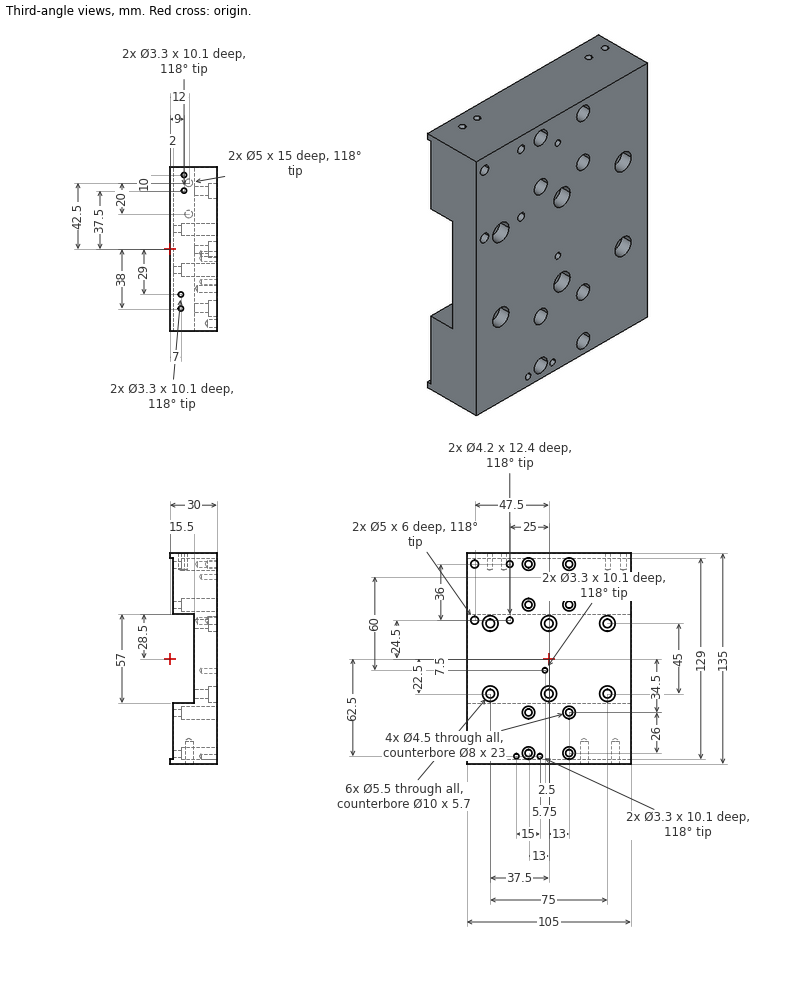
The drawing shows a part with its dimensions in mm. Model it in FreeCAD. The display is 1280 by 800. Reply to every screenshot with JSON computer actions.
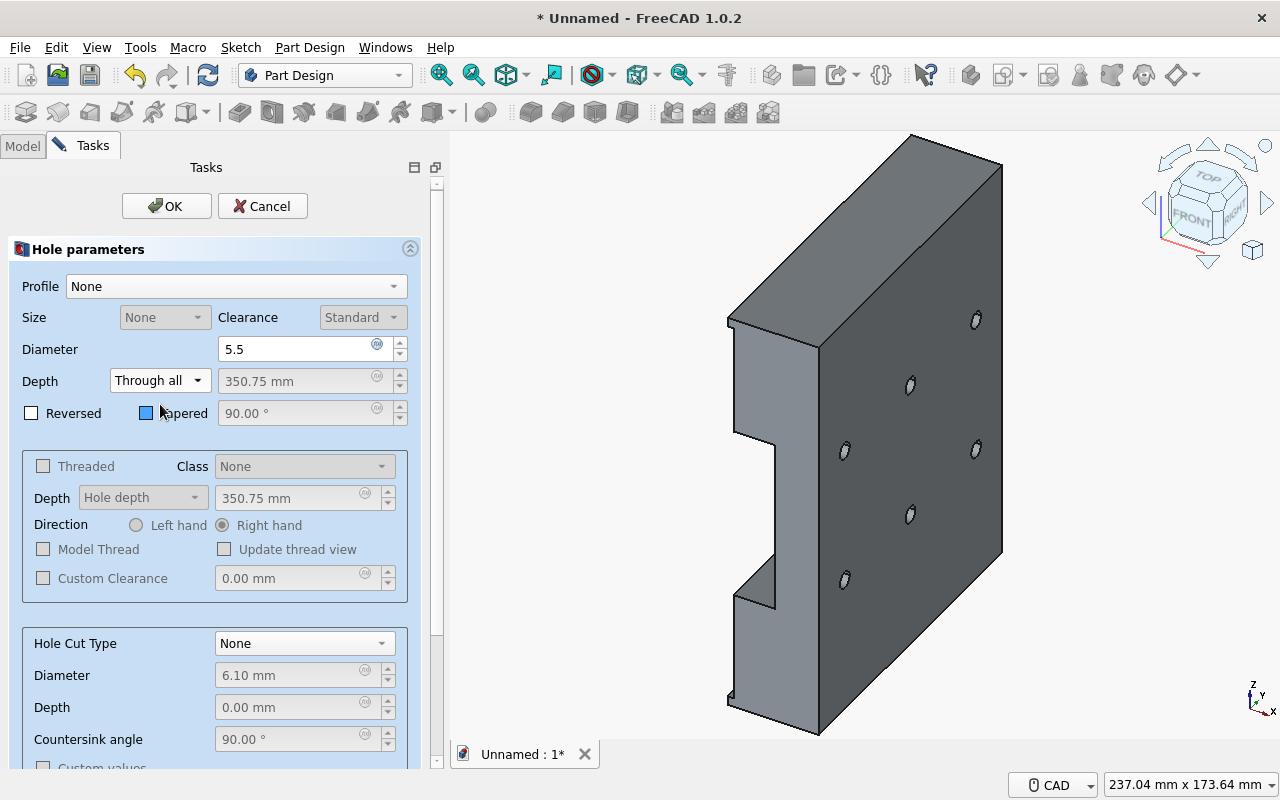
{"action": "left_click", "coordinate": [306, 644]}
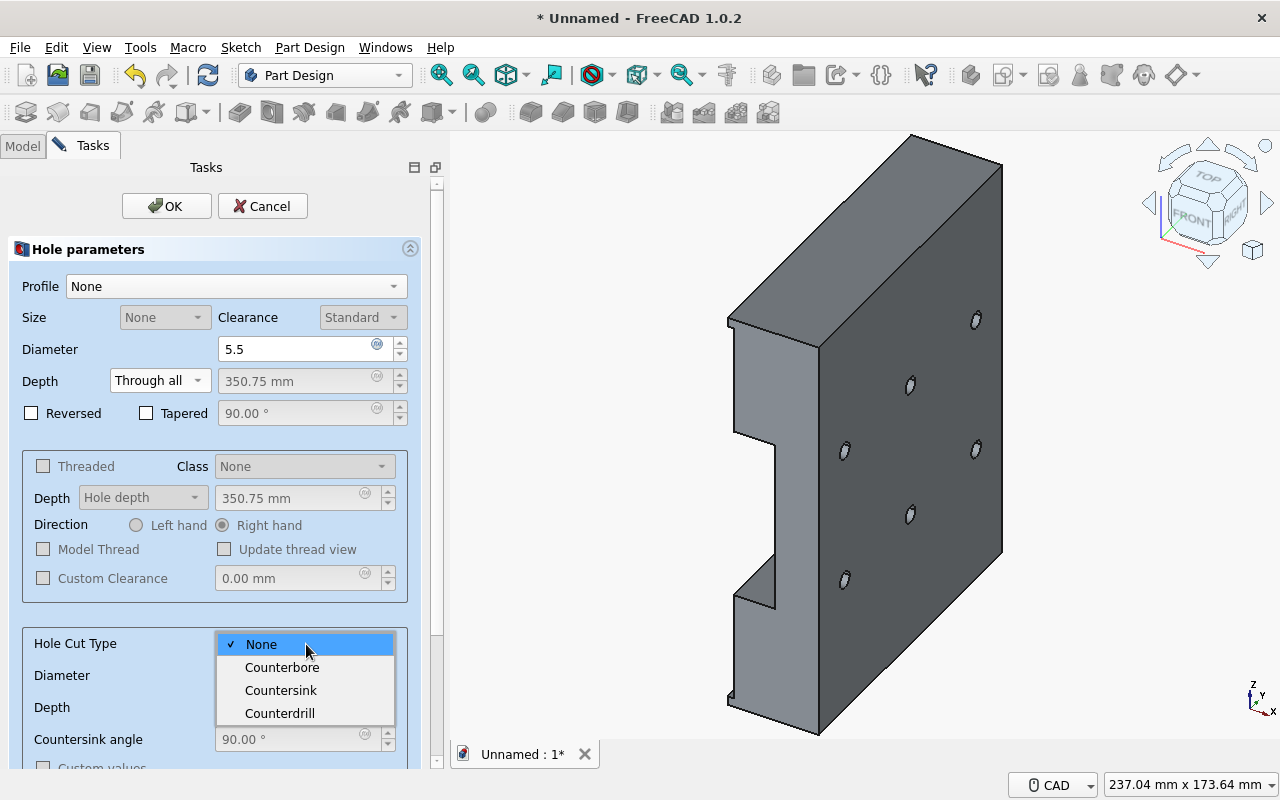
{"action": "left_click", "coordinate": [304, 668]}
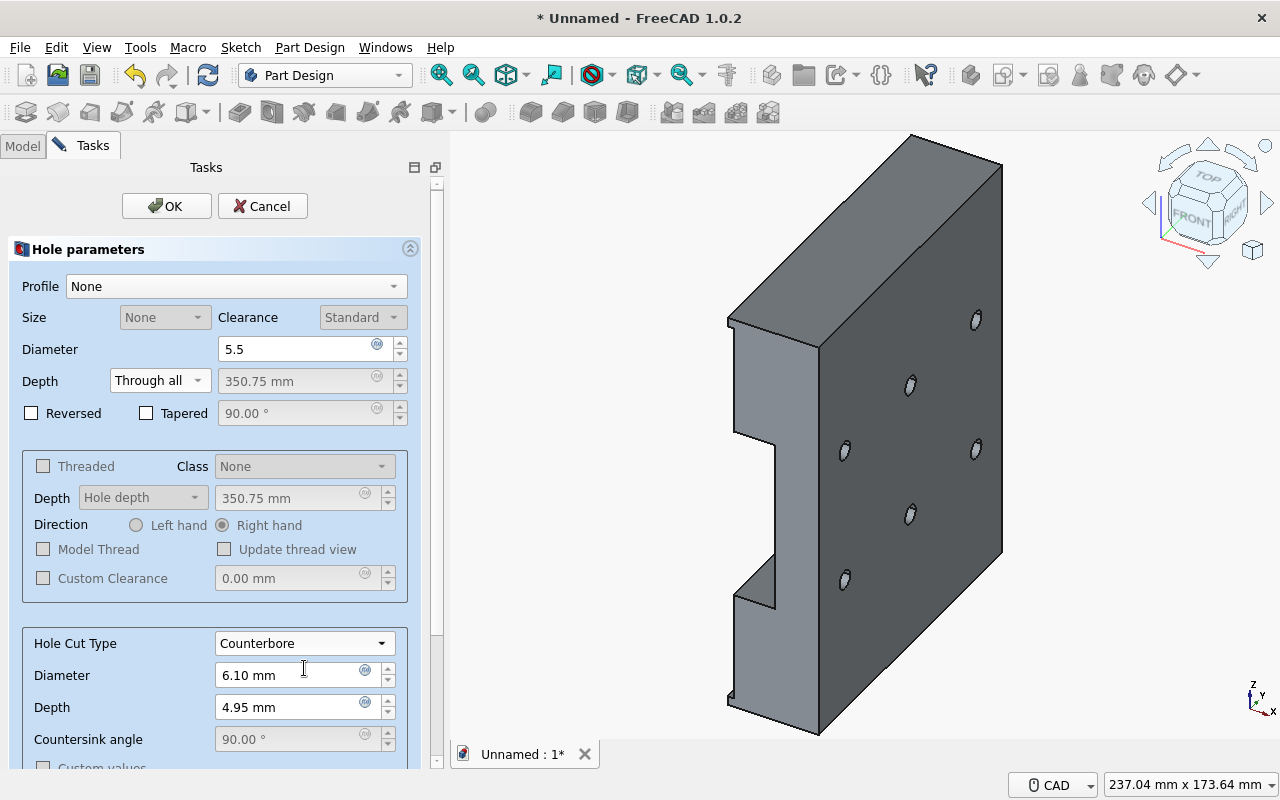
{"action": "triple_click", "coordinate": [298, 675]}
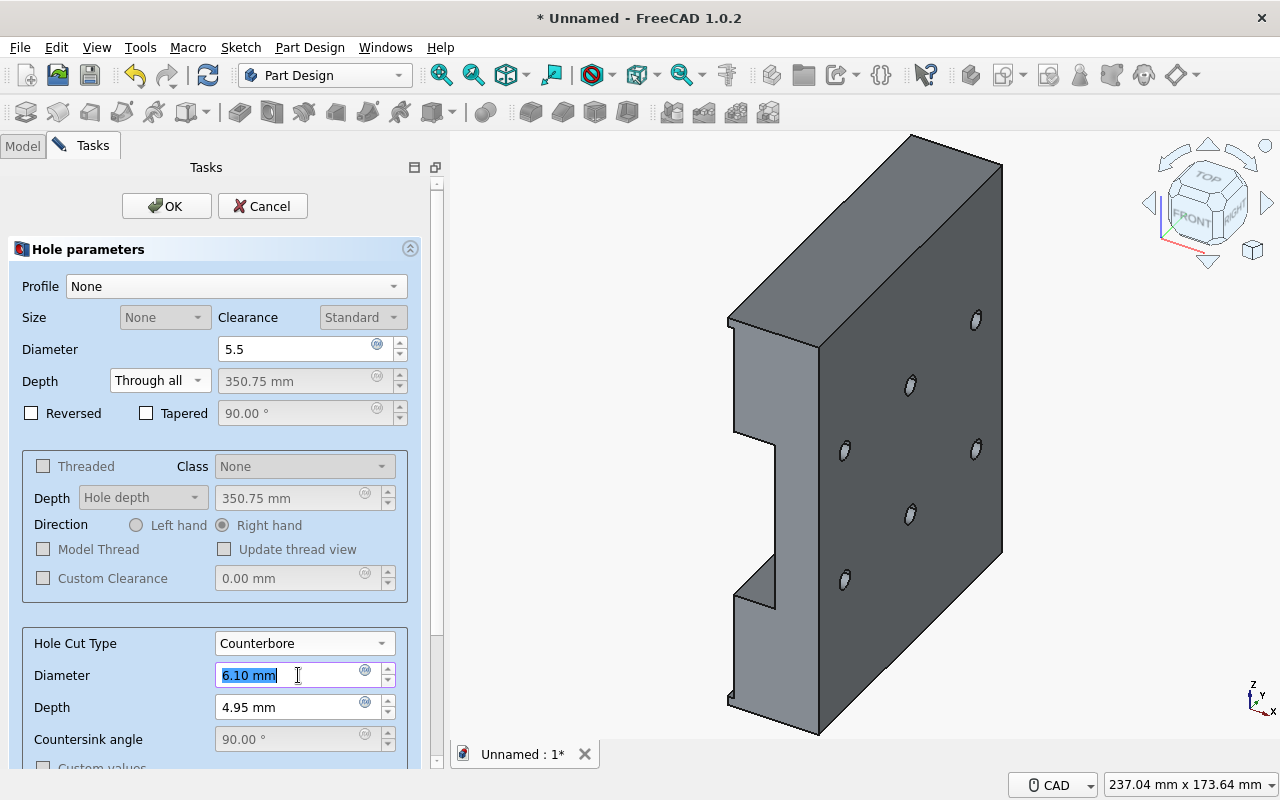
{"action": "type", "text": "10"}
{"action": "key", "text": "Tab"}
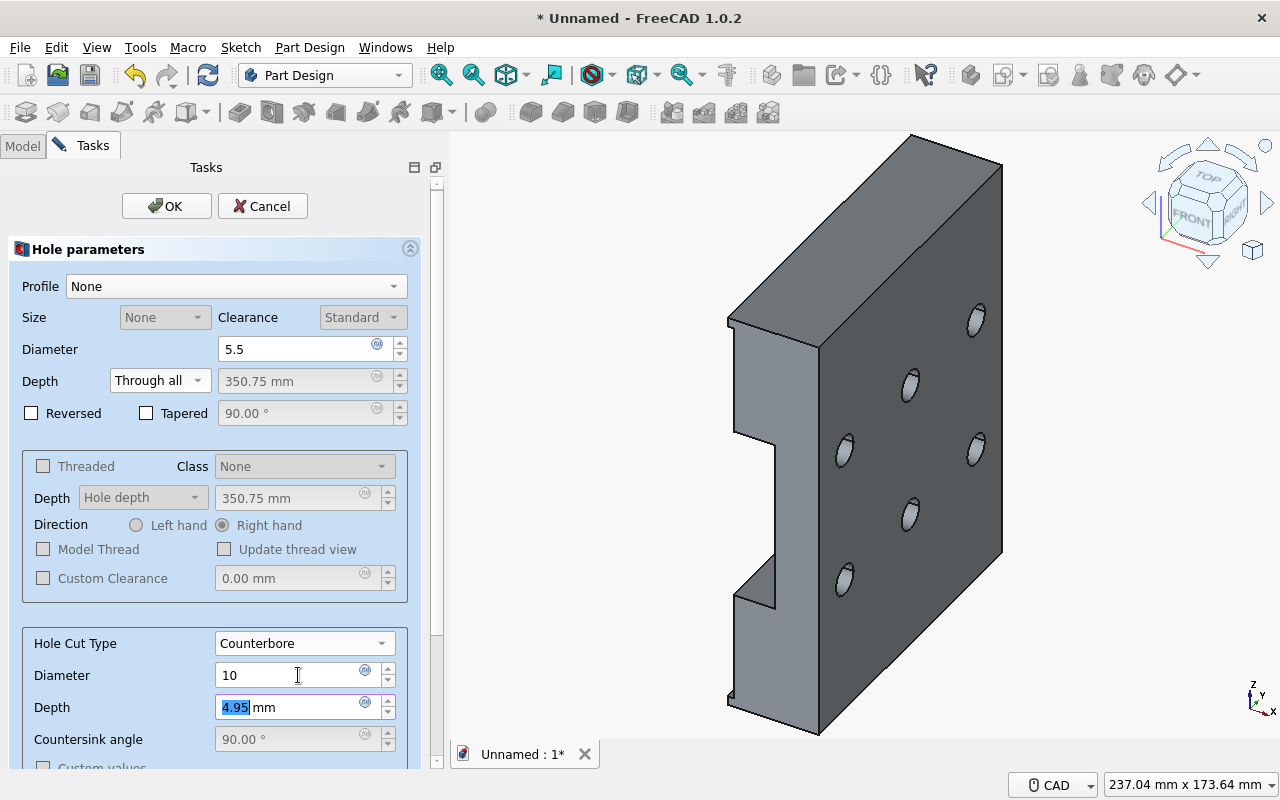
{"action": "type", "text": "5.7"}
{"action": "key", "text": "Tab"}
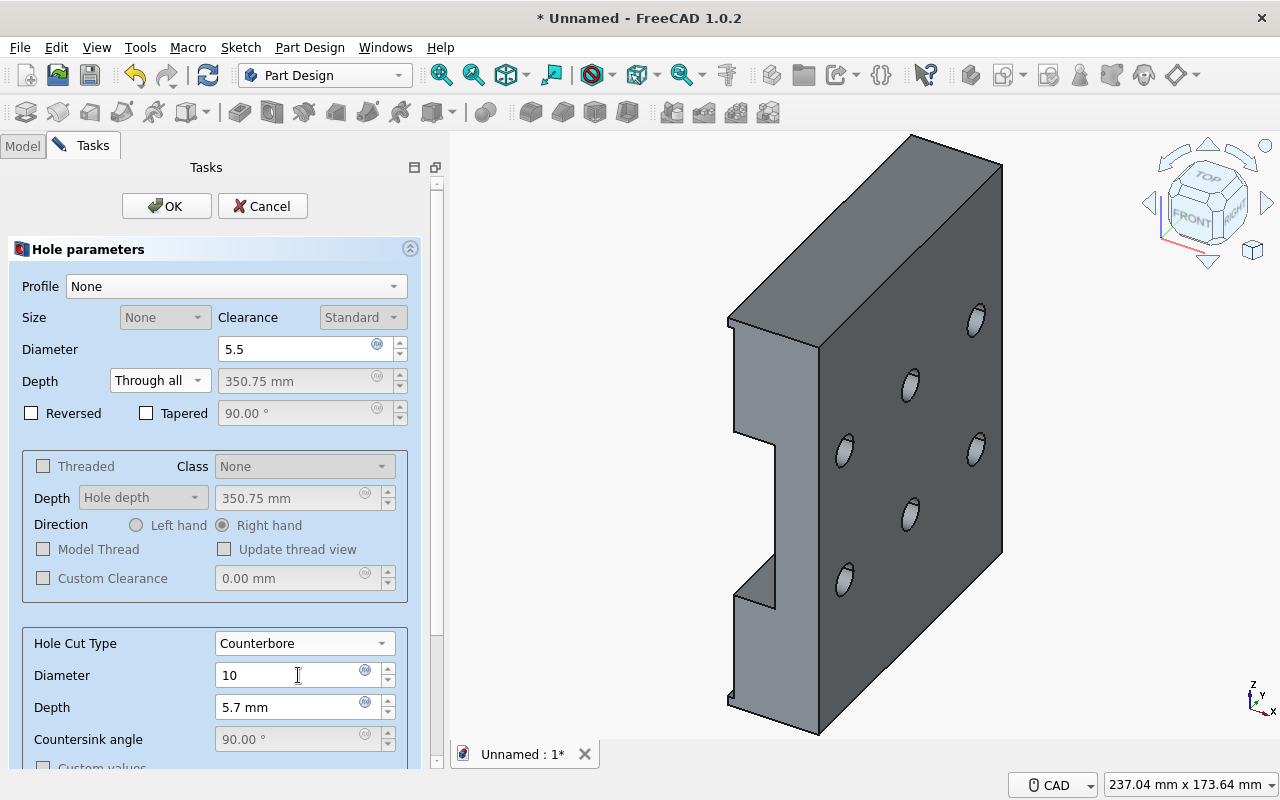
{"action": "left_click", "coordinate": [167, 206]}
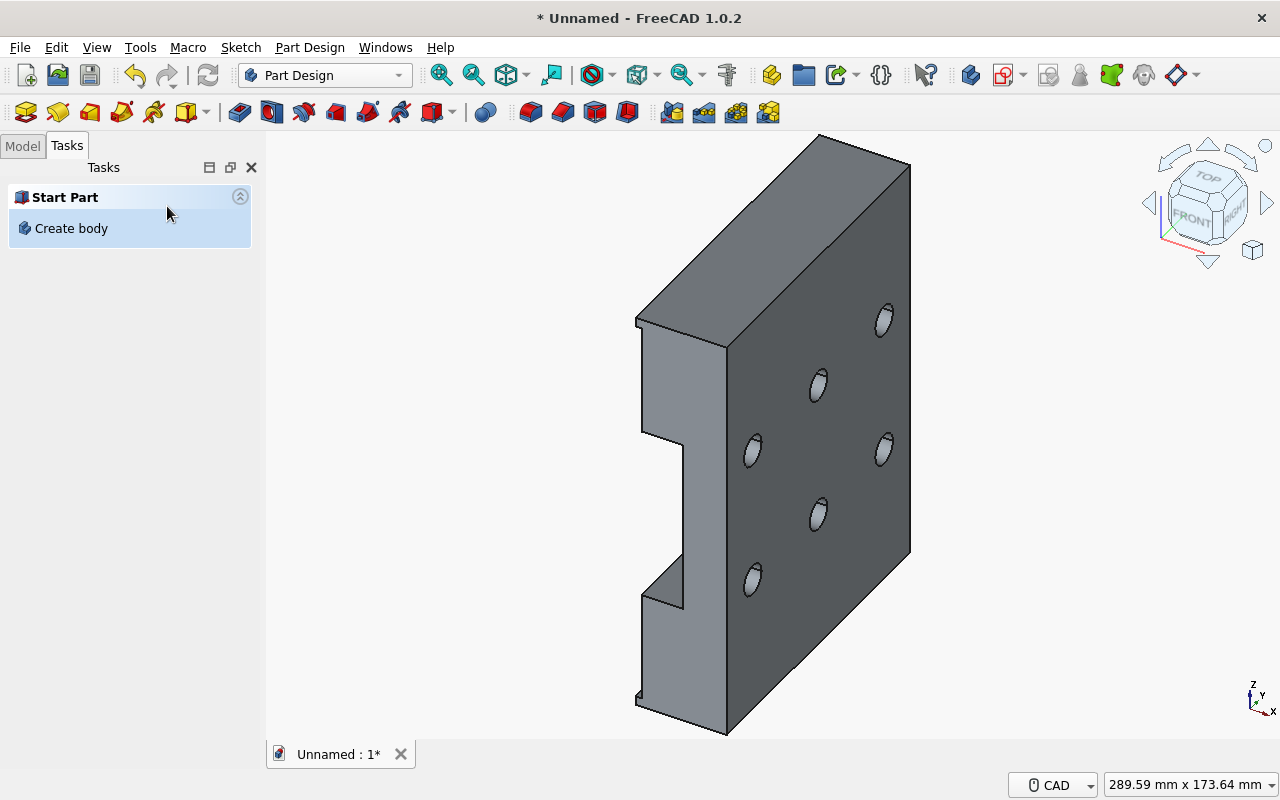
{"action": "left_click", "coordinate": [792, 475]}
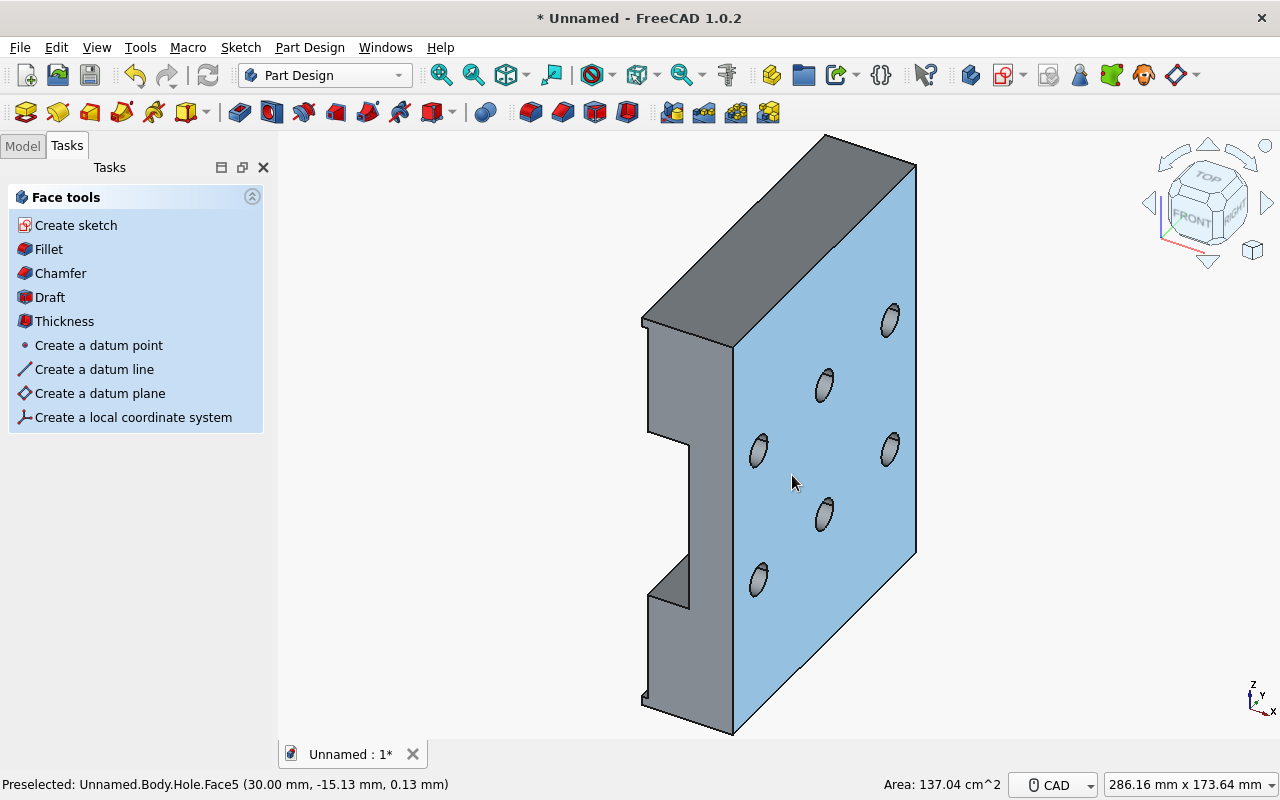
{"action": "left_click", "coordinate": [1004, 76]}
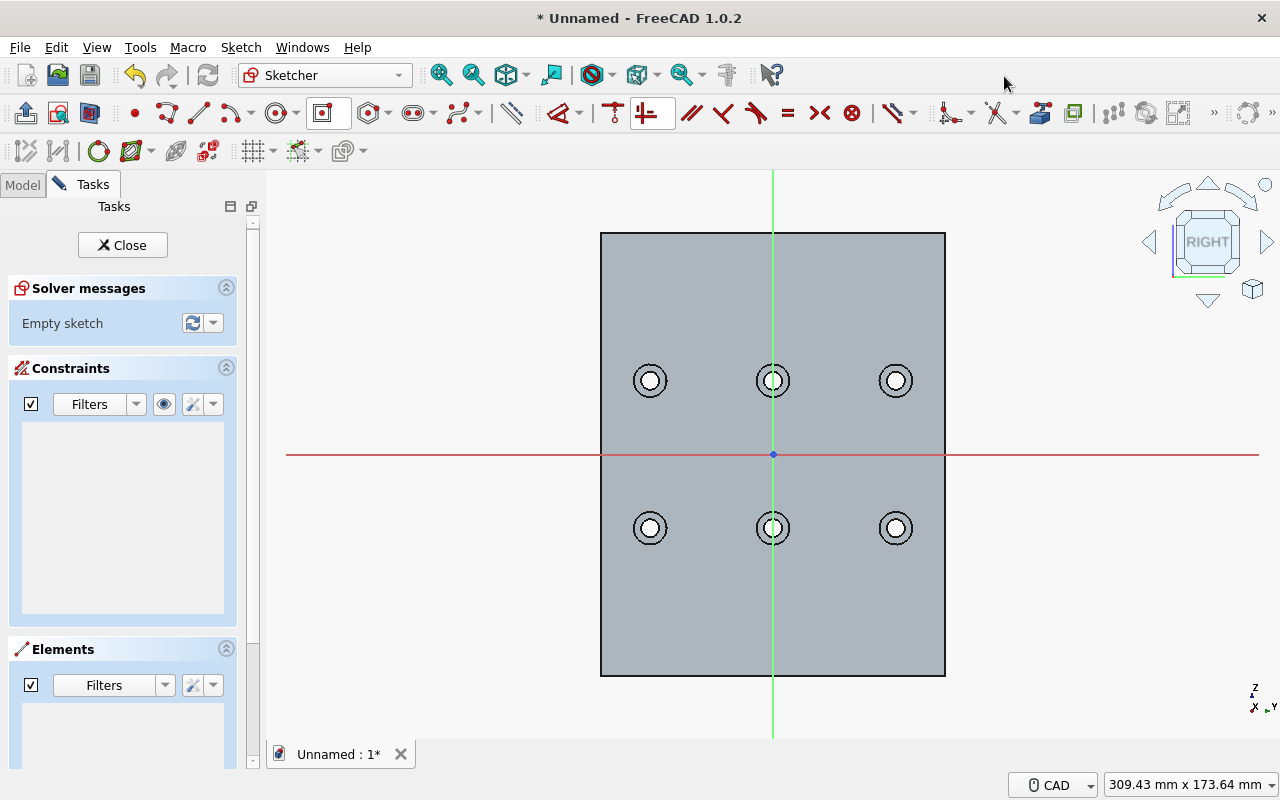
{"action": "scroll", "coordinate": [856, 682], "scroll_direction": "up", "scroll_amount": 3}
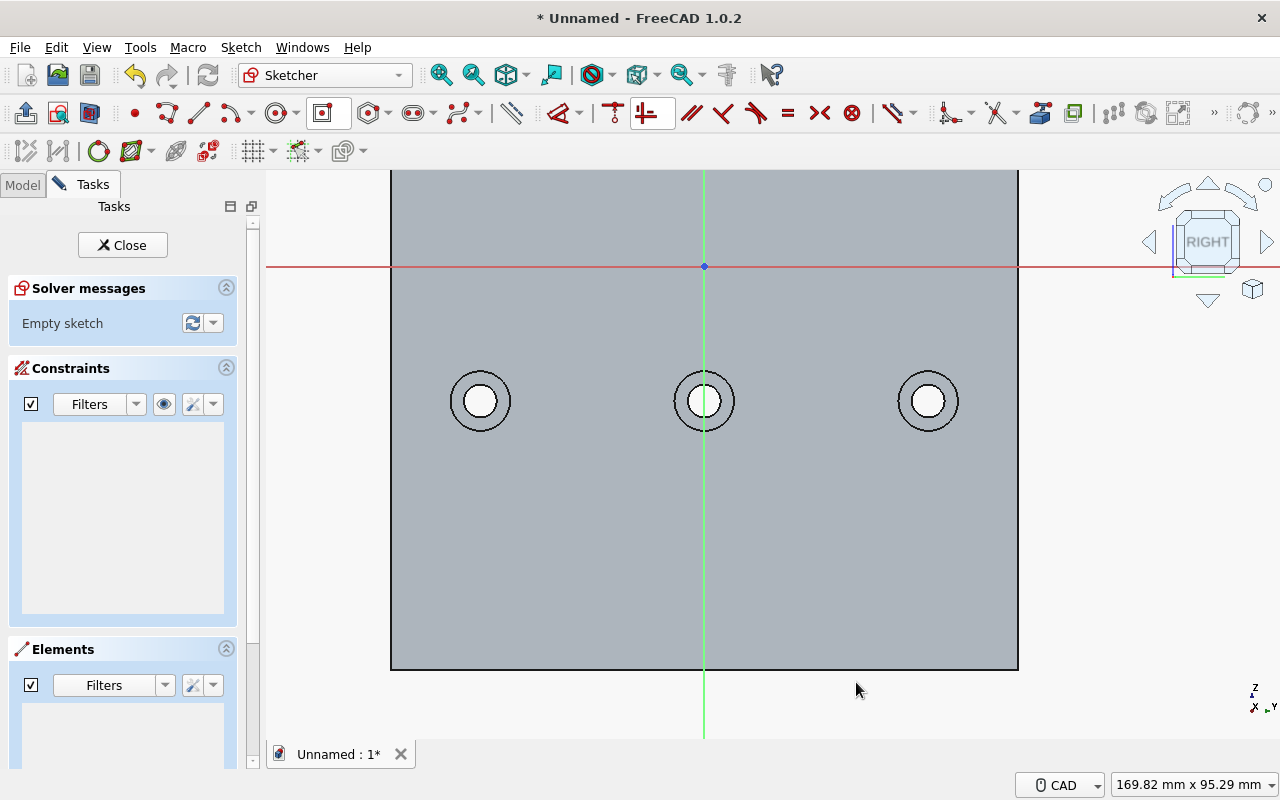
{"action": "left_click", "coordinate": [276, 114]}